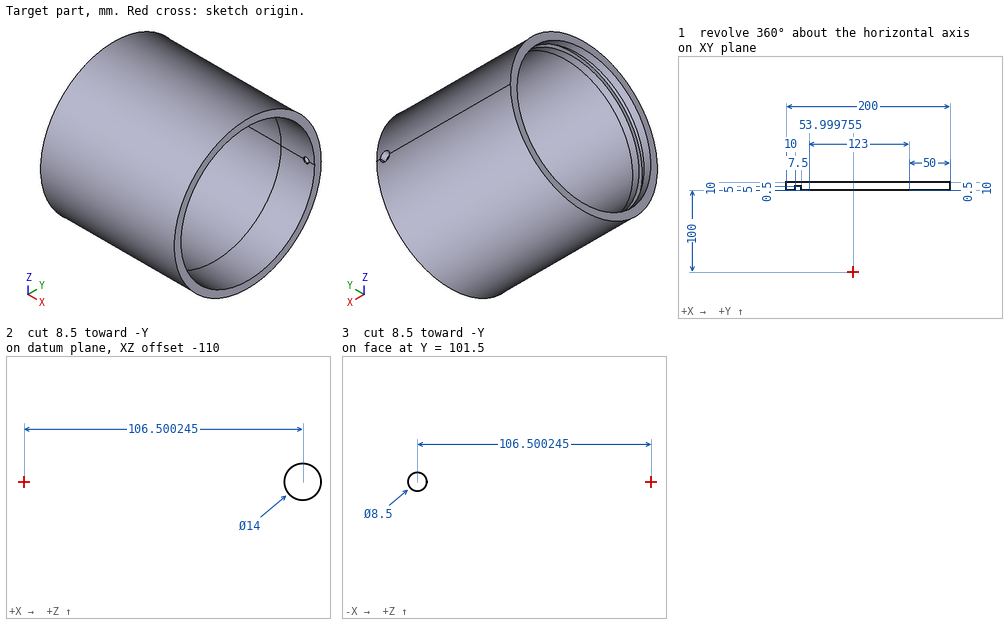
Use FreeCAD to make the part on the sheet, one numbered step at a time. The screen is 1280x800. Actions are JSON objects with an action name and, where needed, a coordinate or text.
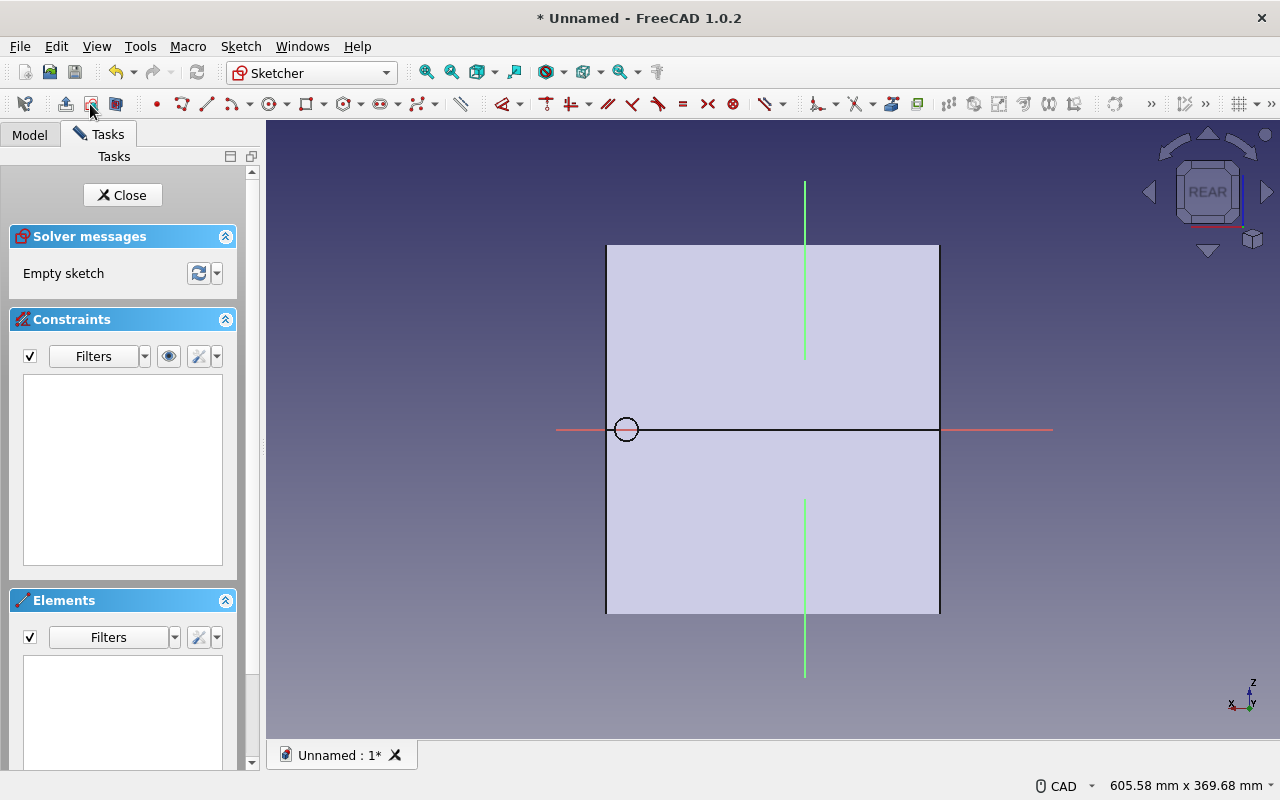
{"action": "scroll", "coordinate": [622, 430], "scroll_direction": "up", "scroll_amount": 15}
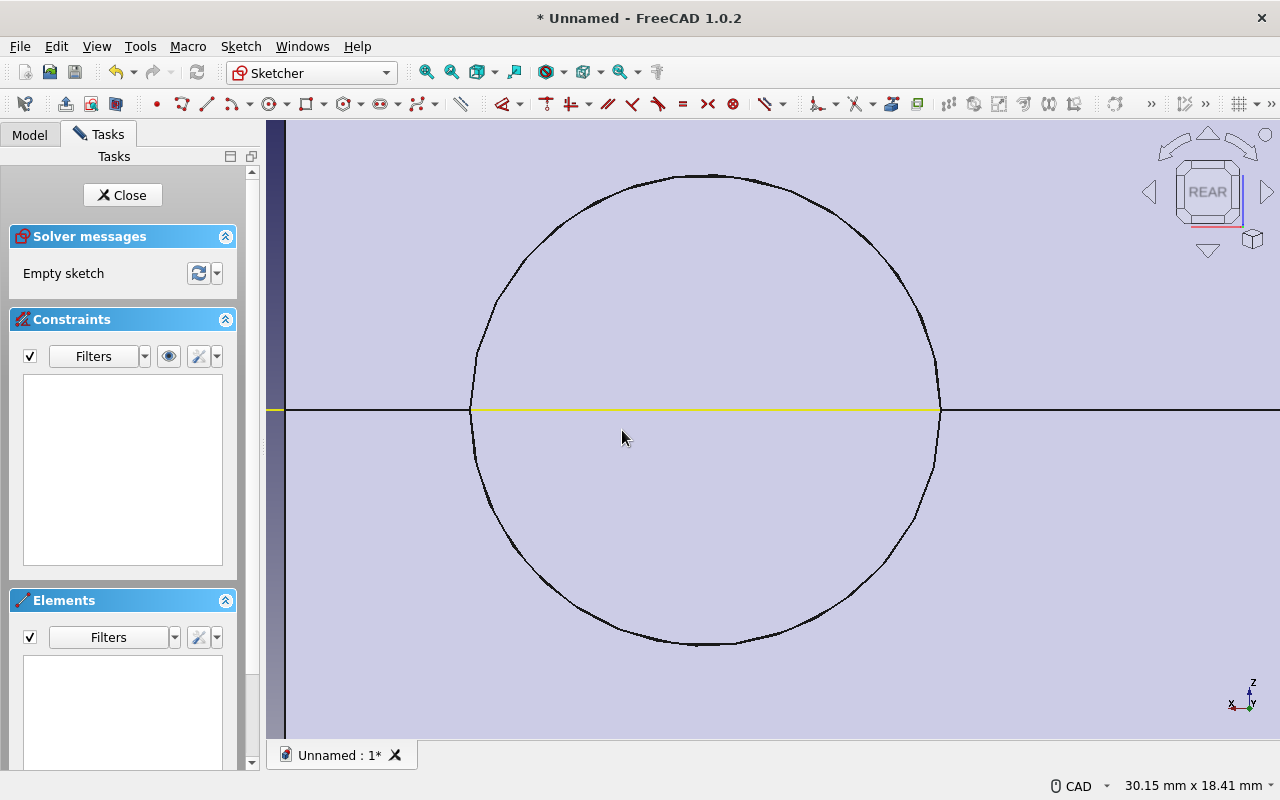
{"action": "scroll", "coordinate": [707, 372], "scroll_direction": "up", "scroll_amount": 2}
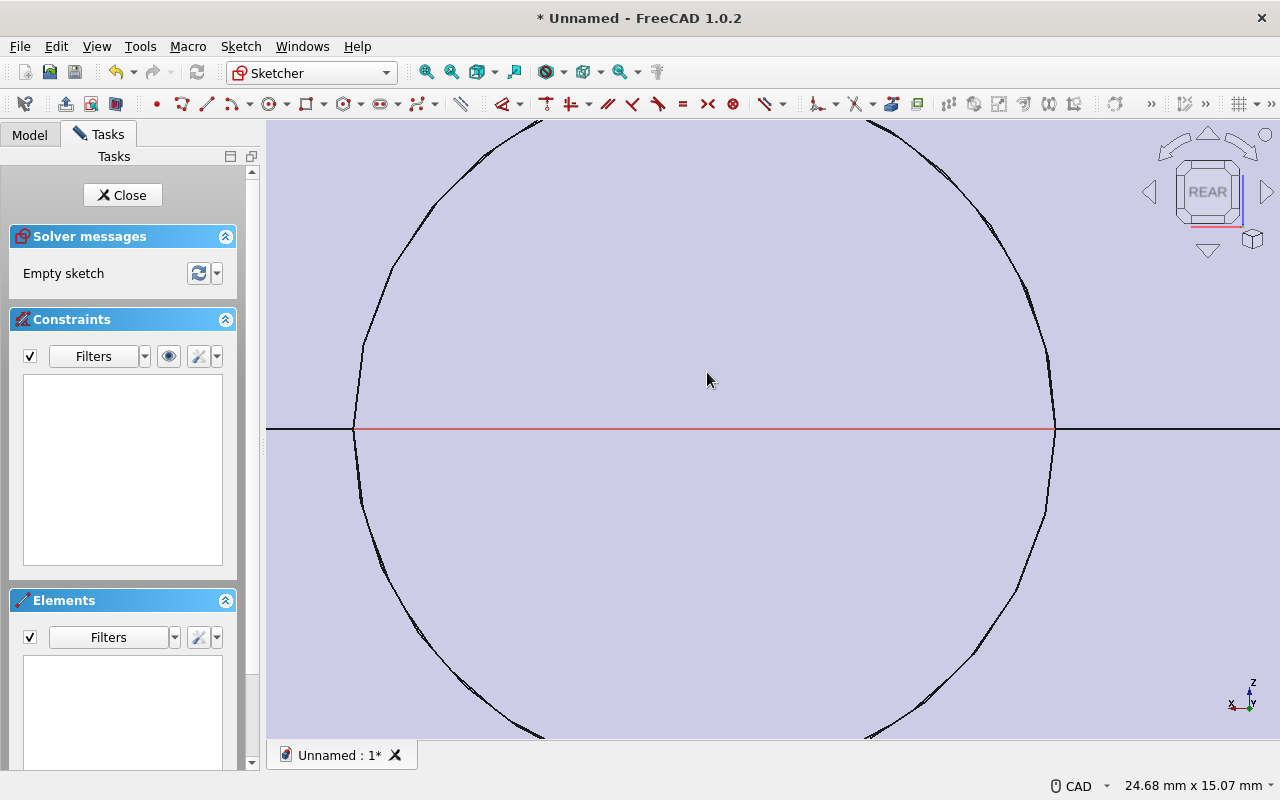
{"action": "key", "text": "g c"}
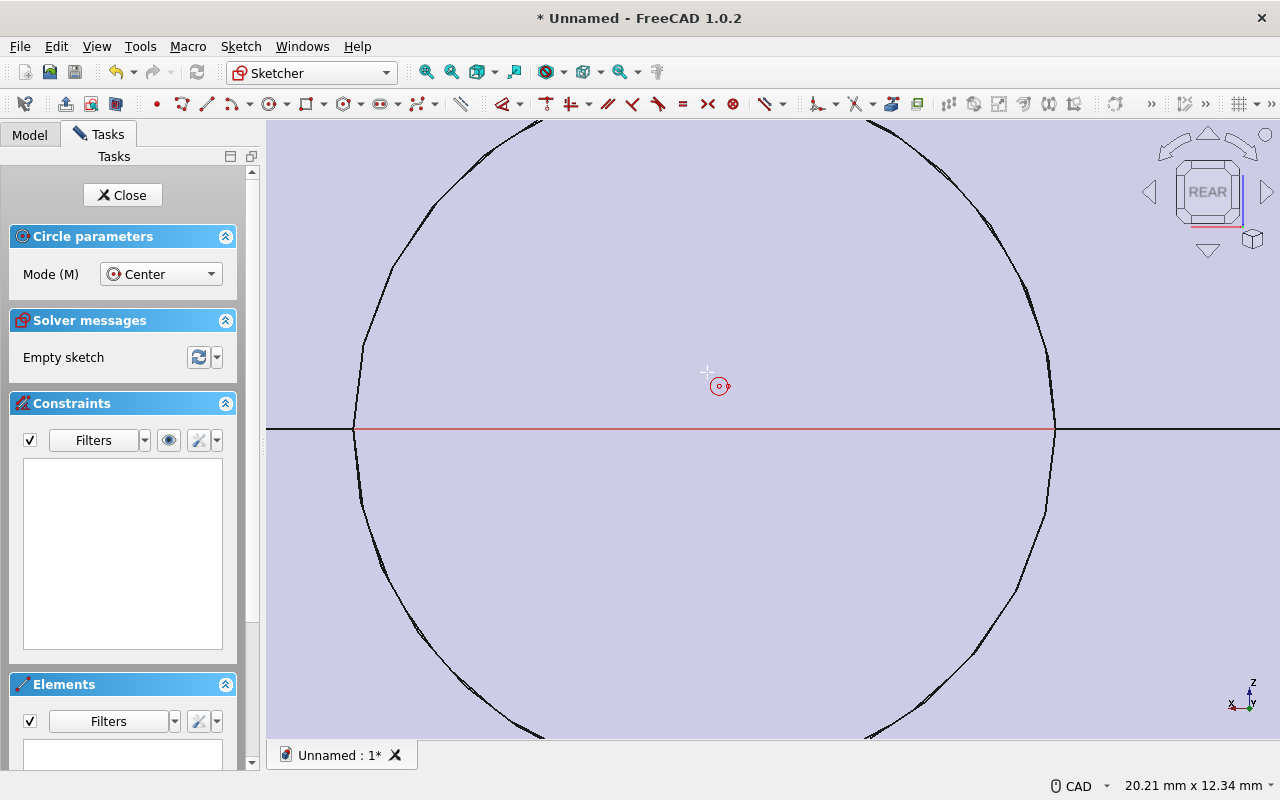
{"action": "left_click", "coordinate": [704, 429]}
{"action": "mouse_move", "coordinate": [855, 278]}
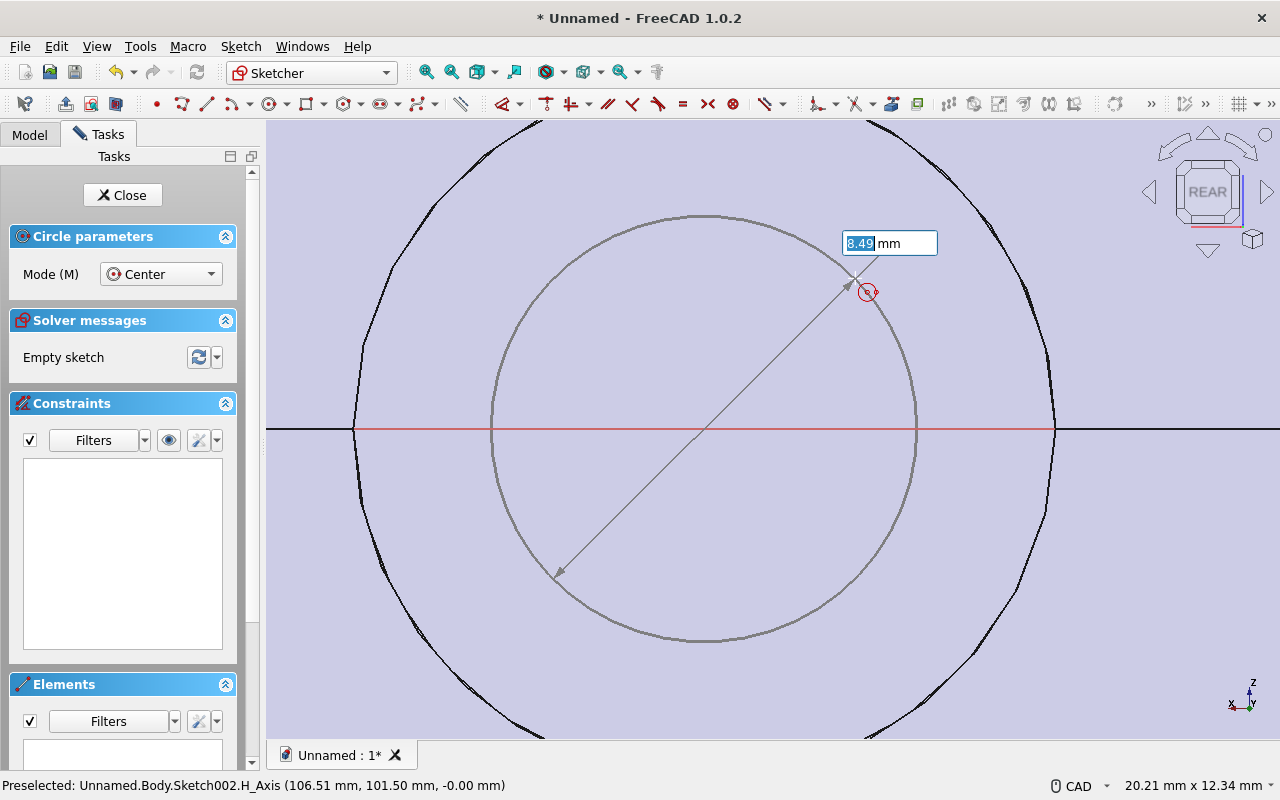
{"action": "type", "text": "8.5"}
{"action": "key", "text": "Return"}
{"action": "key", "text": "Escape"}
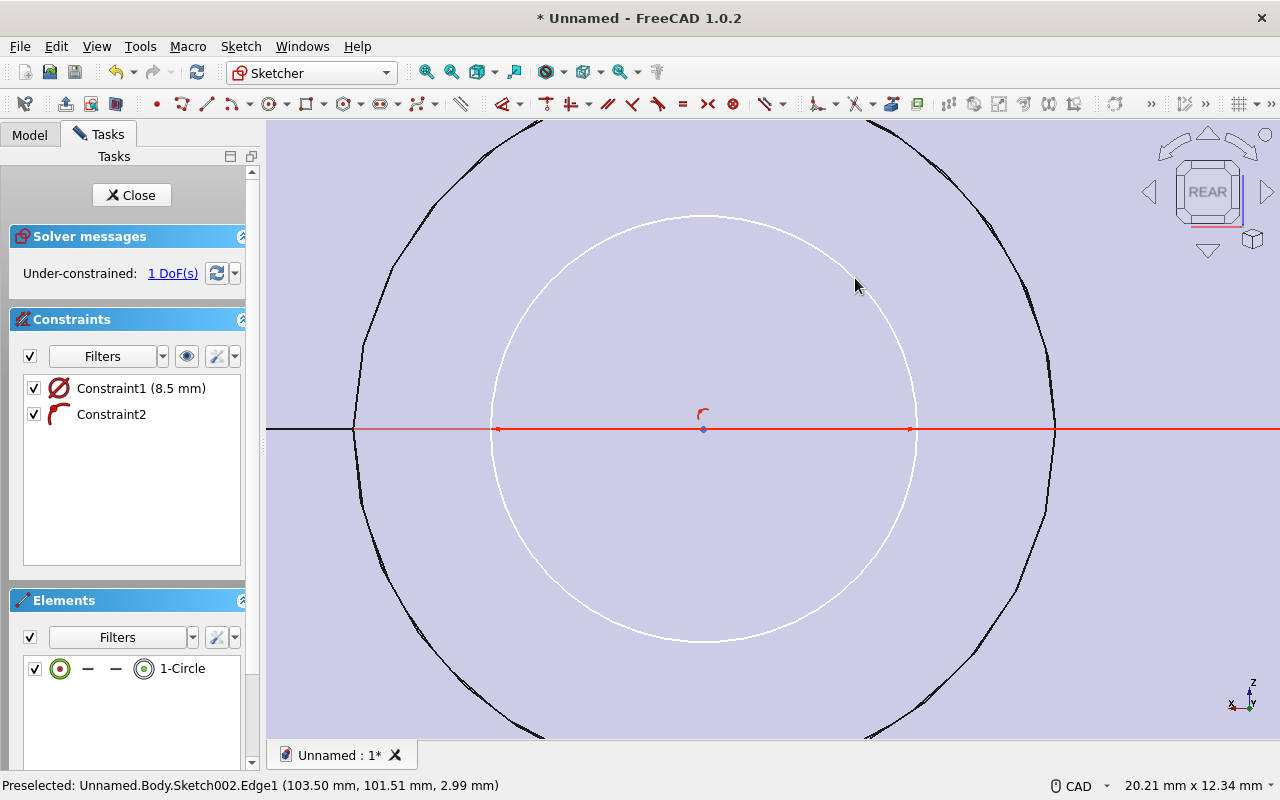
{"action": "key", "text": "d"}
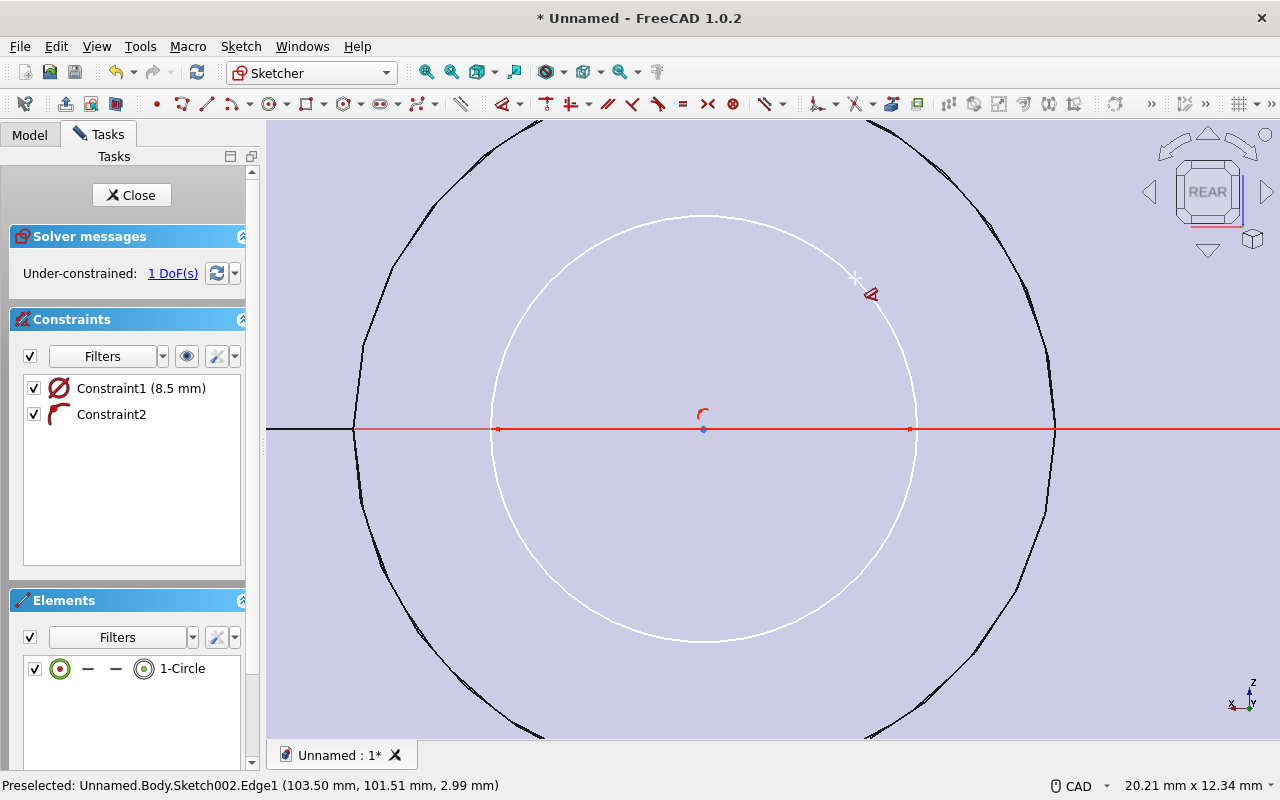
{"action": "left_click", "coordinate": [704, 429]}
{"action": "left_click", "coordinate": [815, 463]}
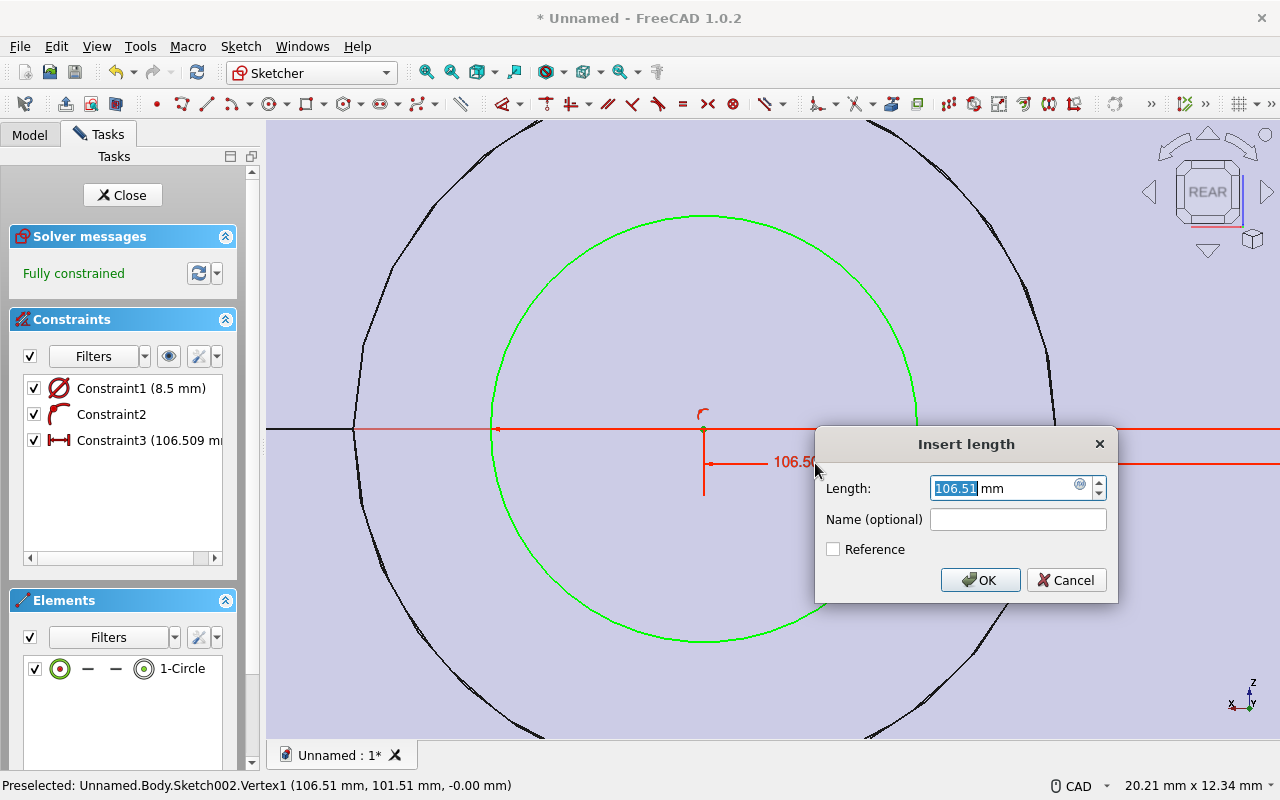
{"action": "type", "text": "106.500245"}
{"action": "key", "text": "Return"}
{"action": "key", "text": "Escape"}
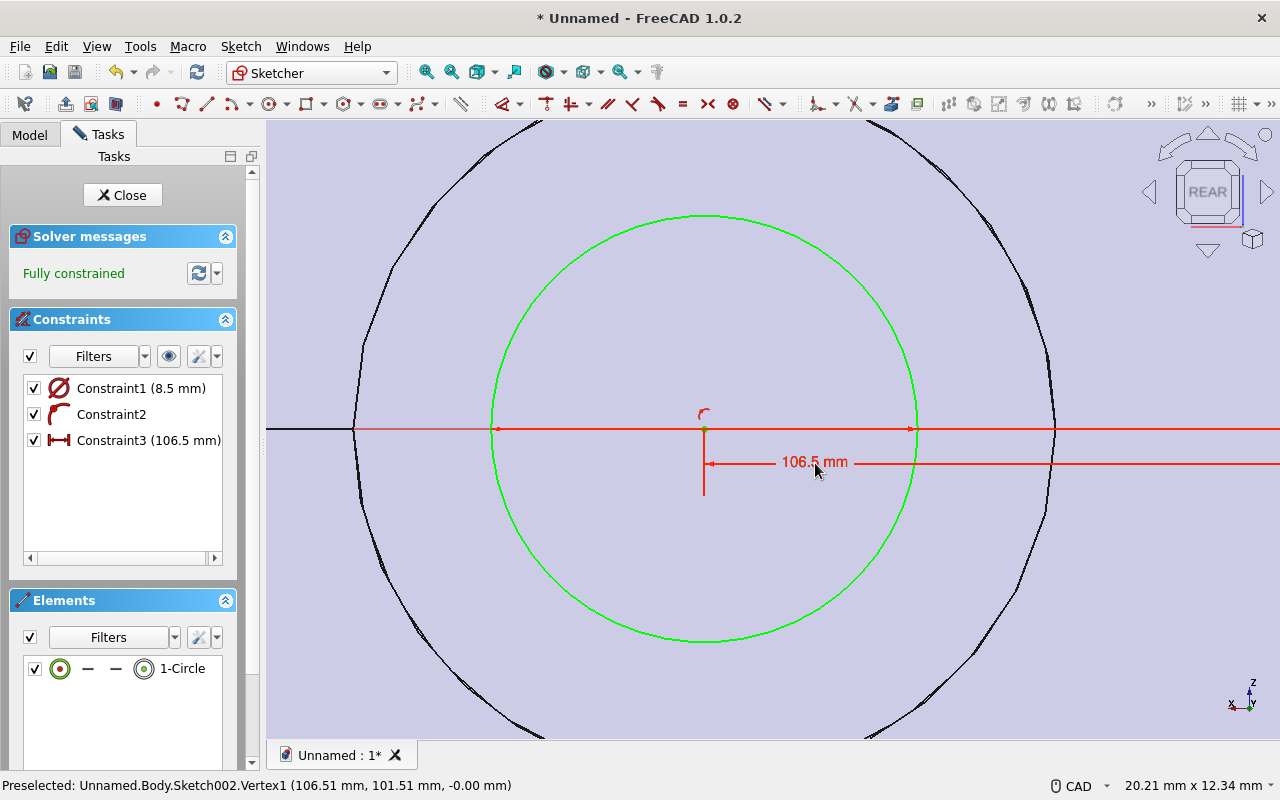
{"action": "left_click", "coordinate": [123, 195]}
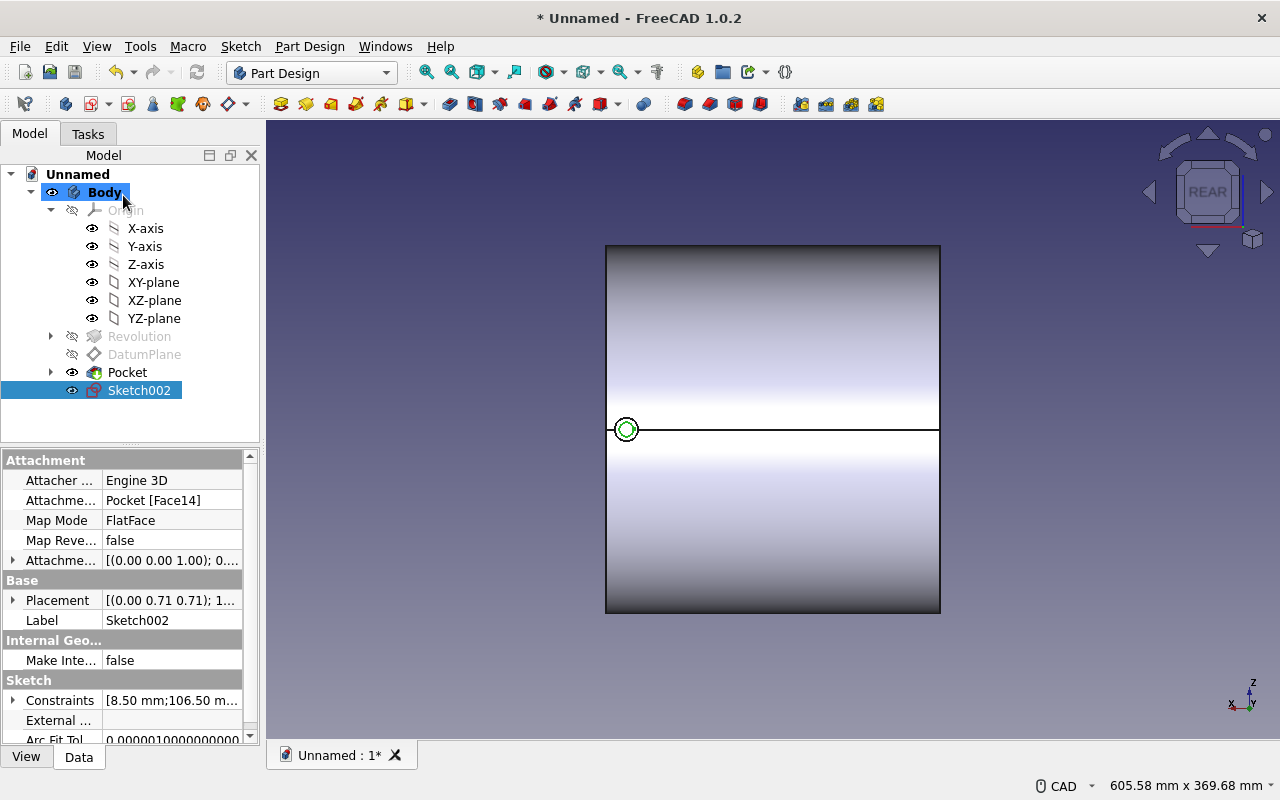
{"action": "left_click", "coordinate": [450, 104]}